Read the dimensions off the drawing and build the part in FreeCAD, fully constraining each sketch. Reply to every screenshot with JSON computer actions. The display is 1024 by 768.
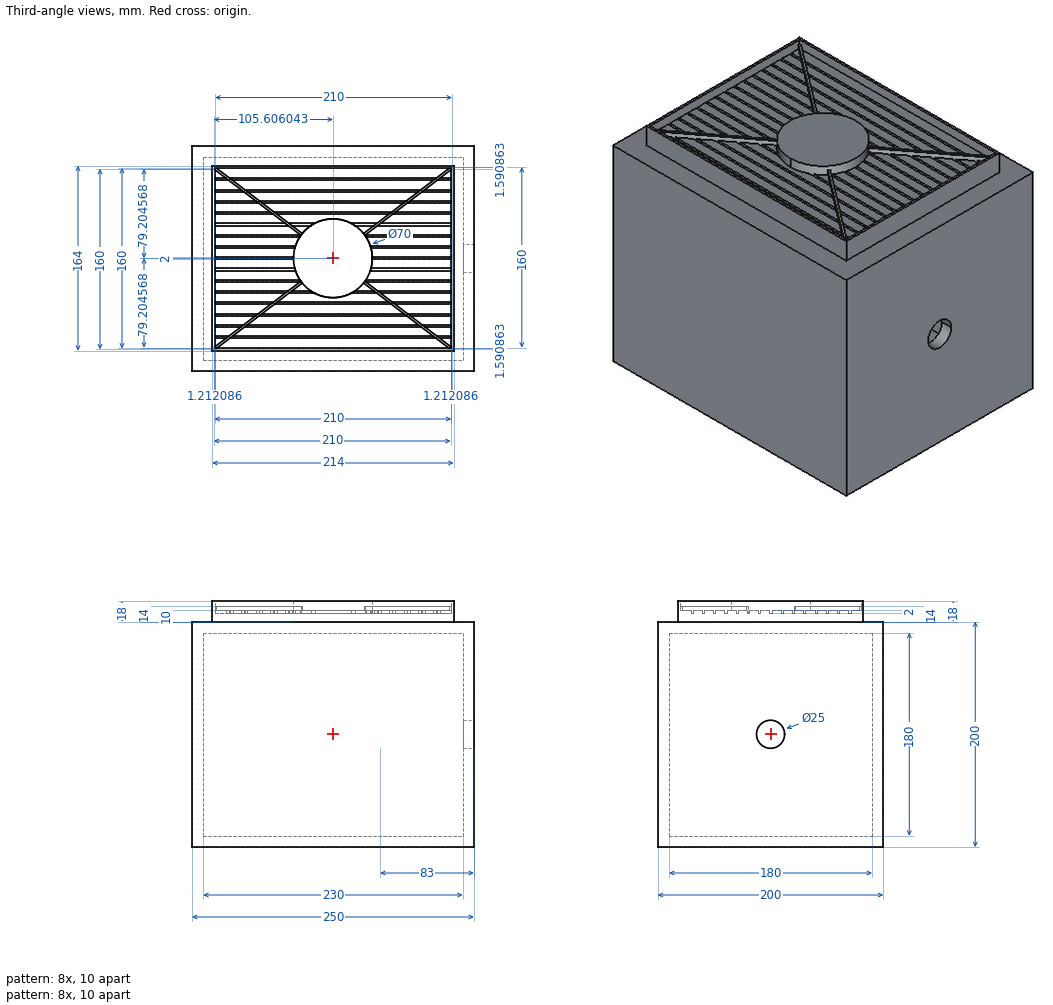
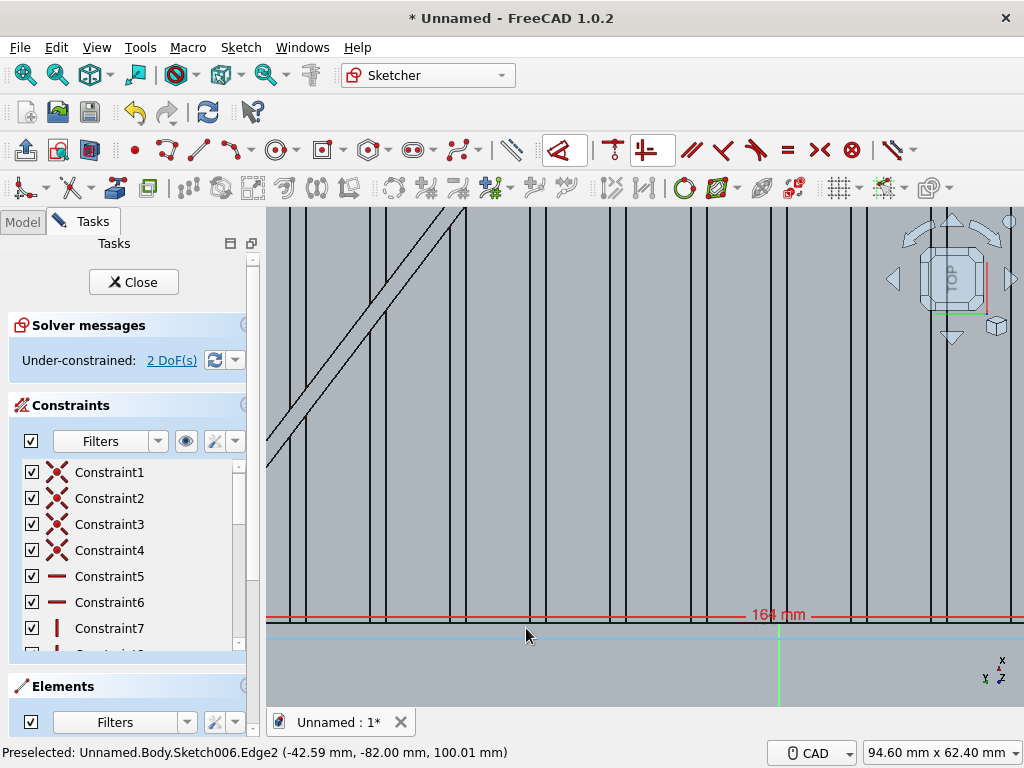
{"action": "left_click", "coordinate": [522, 622]}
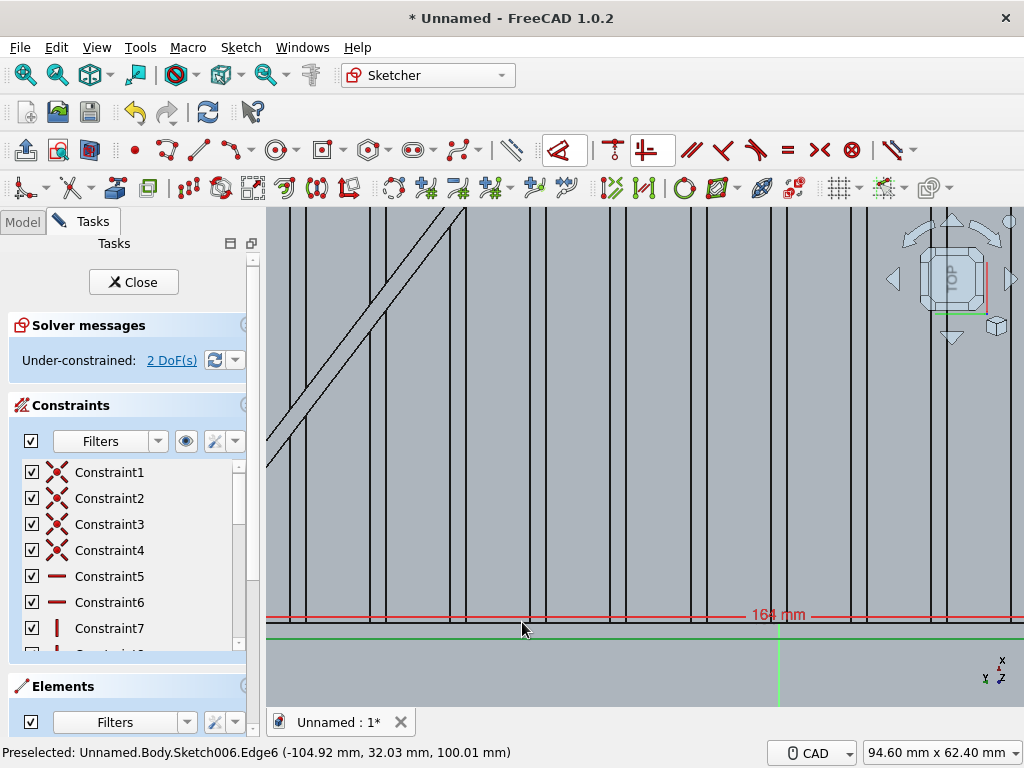
{"action": "left_click", "coordinate": [582, 150]}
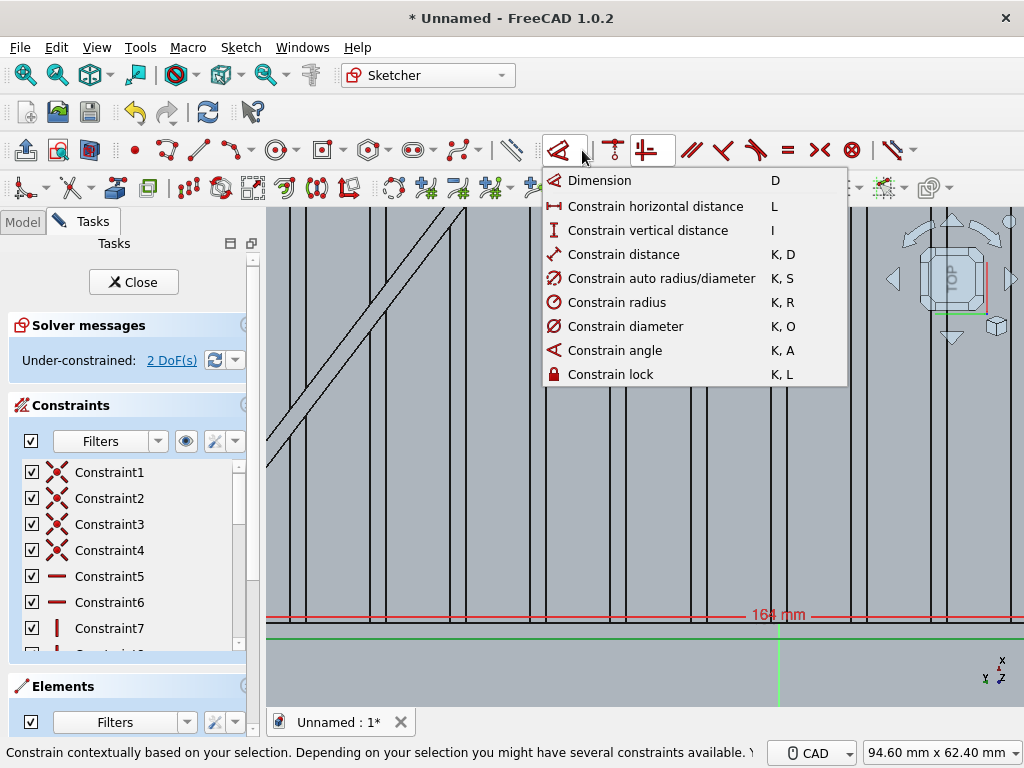
{"action": "left_click", "coordinate": [695, 206]}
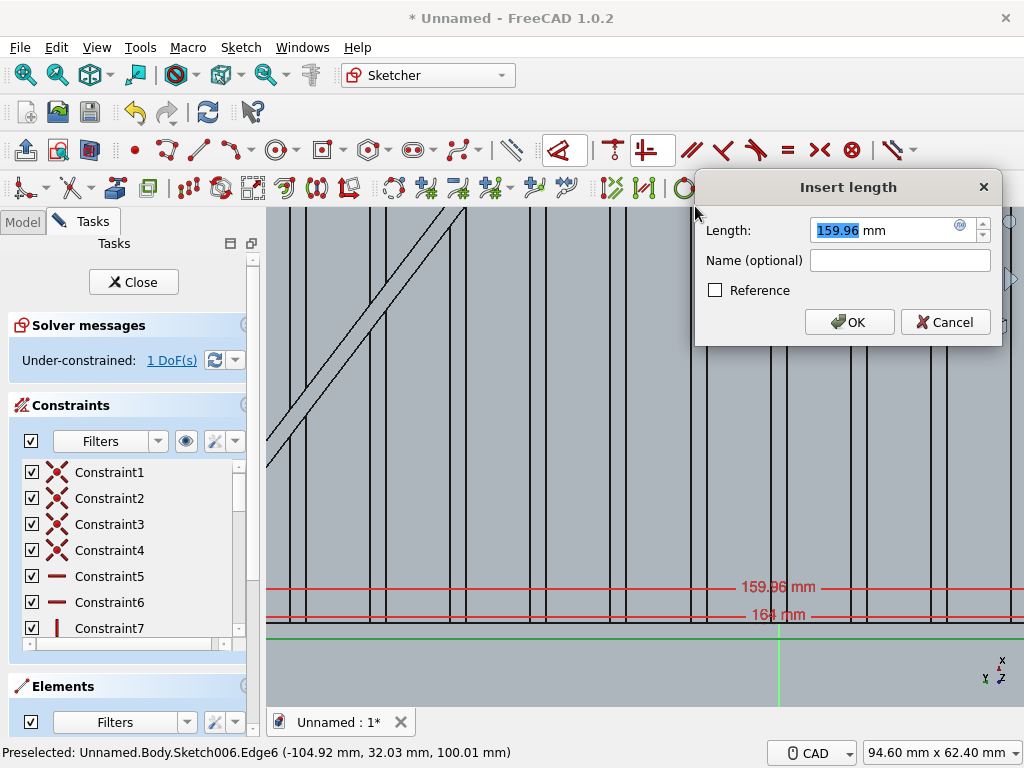
{"action": "type", "text": "160"}
{"action": "key", "text": "Return"}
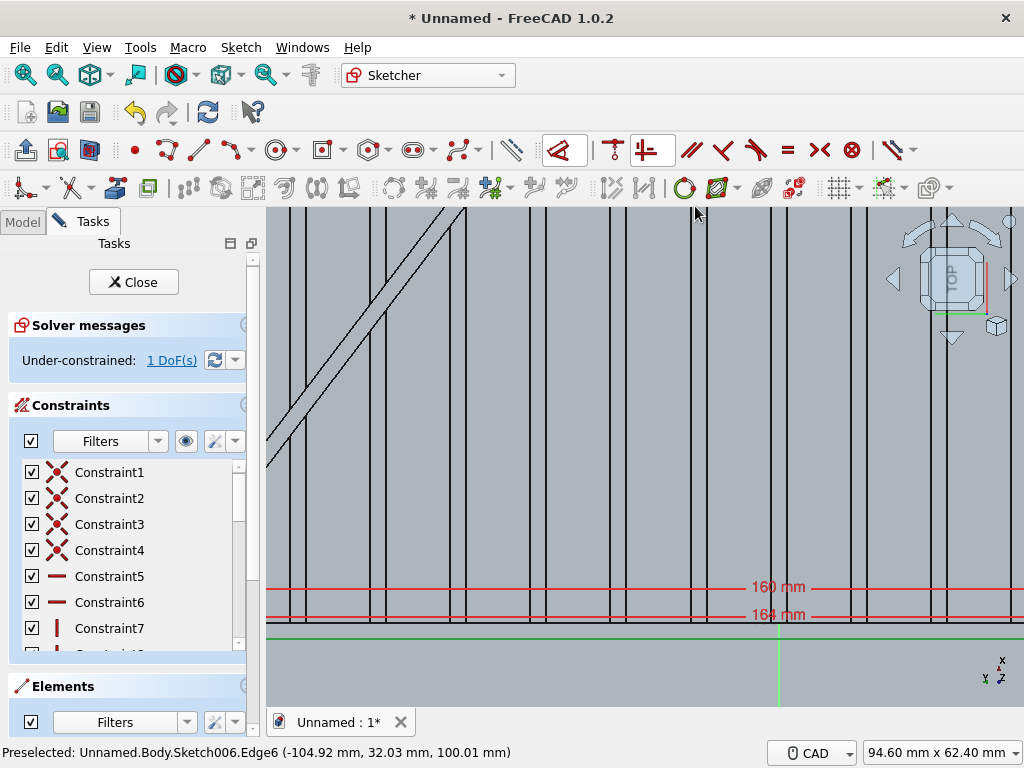
{"action": "scroll", "coordinate": [525, 628], "scroll_direction": "down", "scroll_amount": 8}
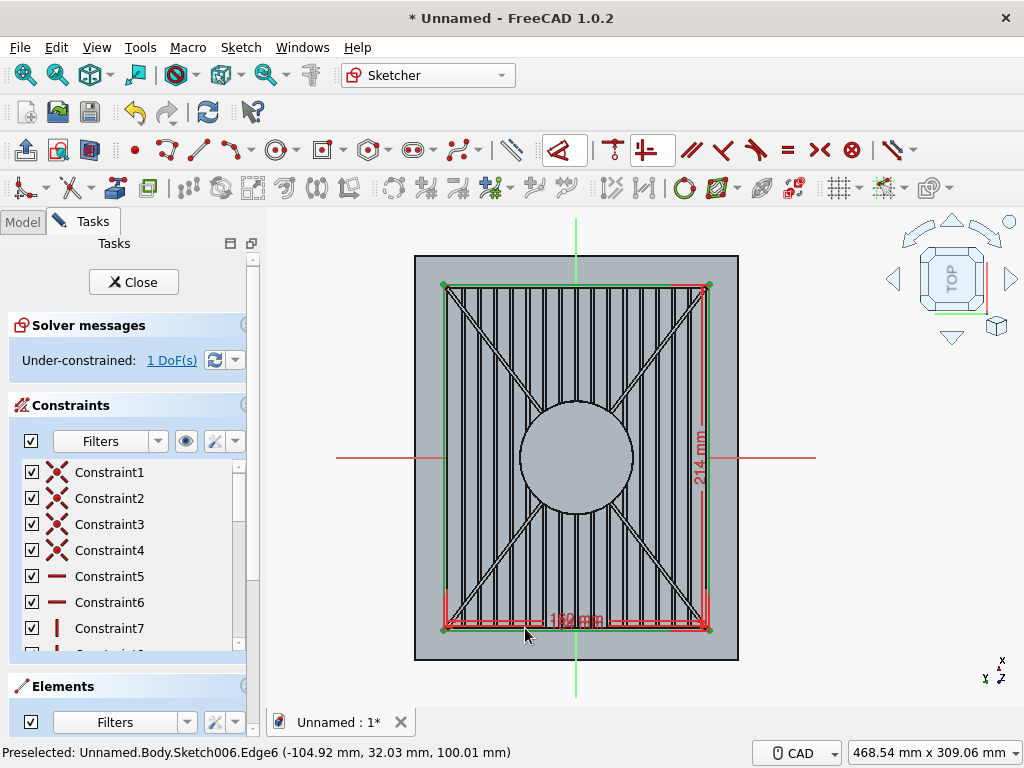
{"action": "scroll", "coordinate": [706, 526], "scroll_direction": "up", "scroll_amount": 8}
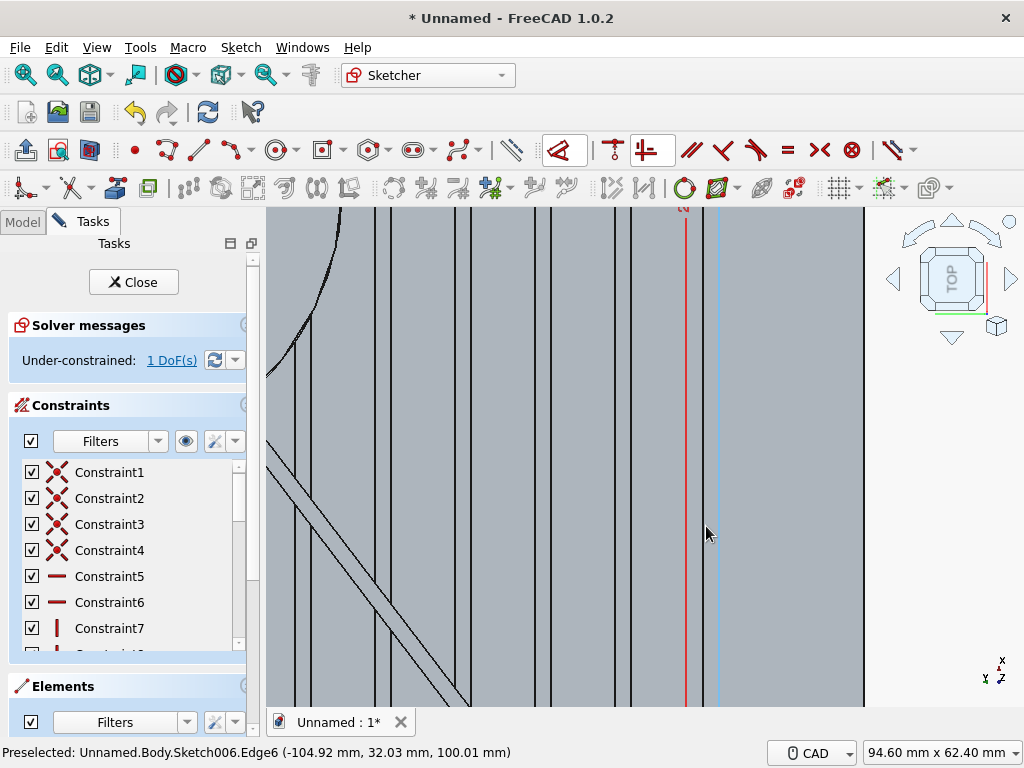
{"action": "left_click", "coordinate": [703, 522]}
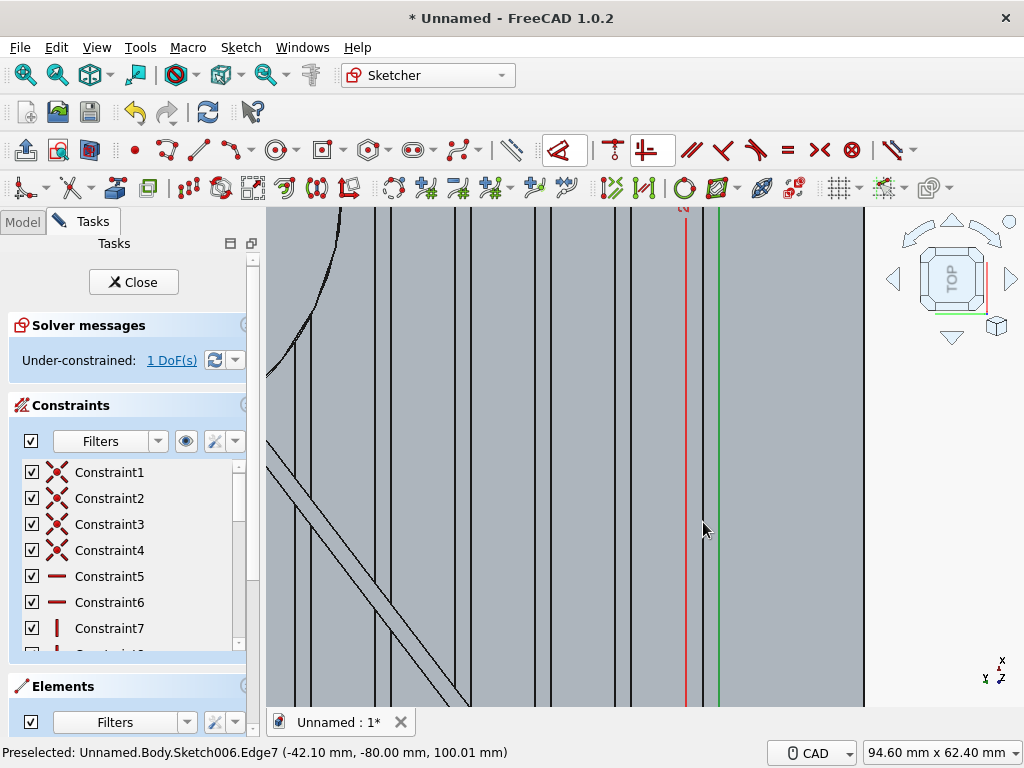
{"action": "key", "text": "i"}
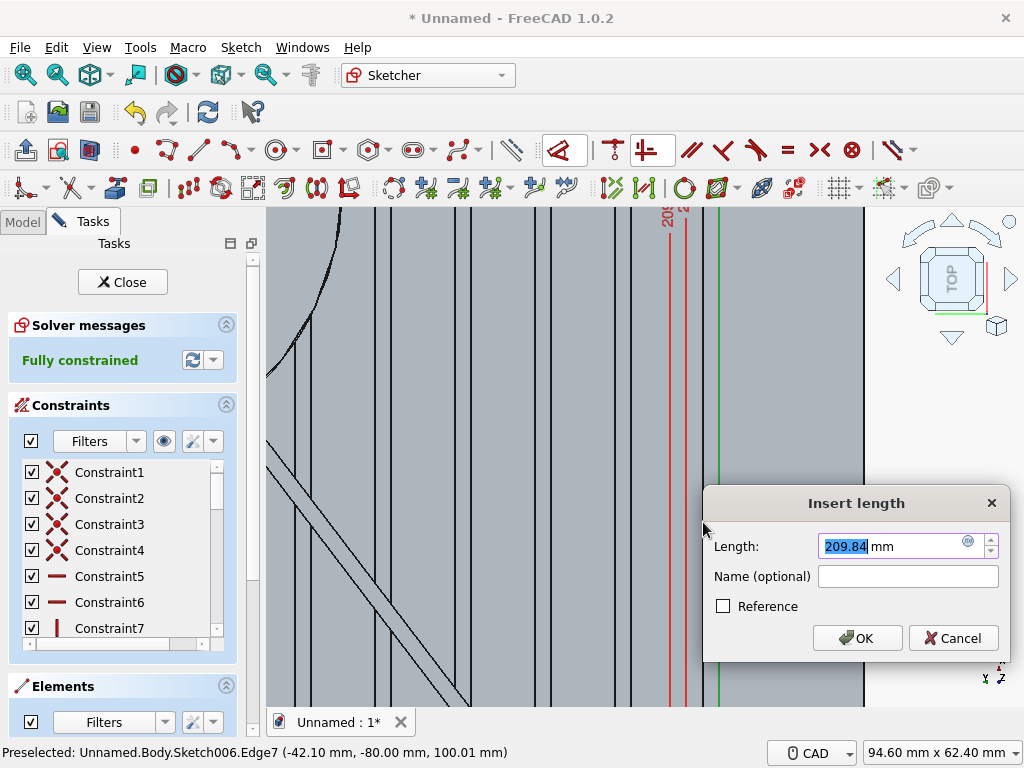
{"action": "type", "text": "210"}
{"action": "key", "text": "Return"}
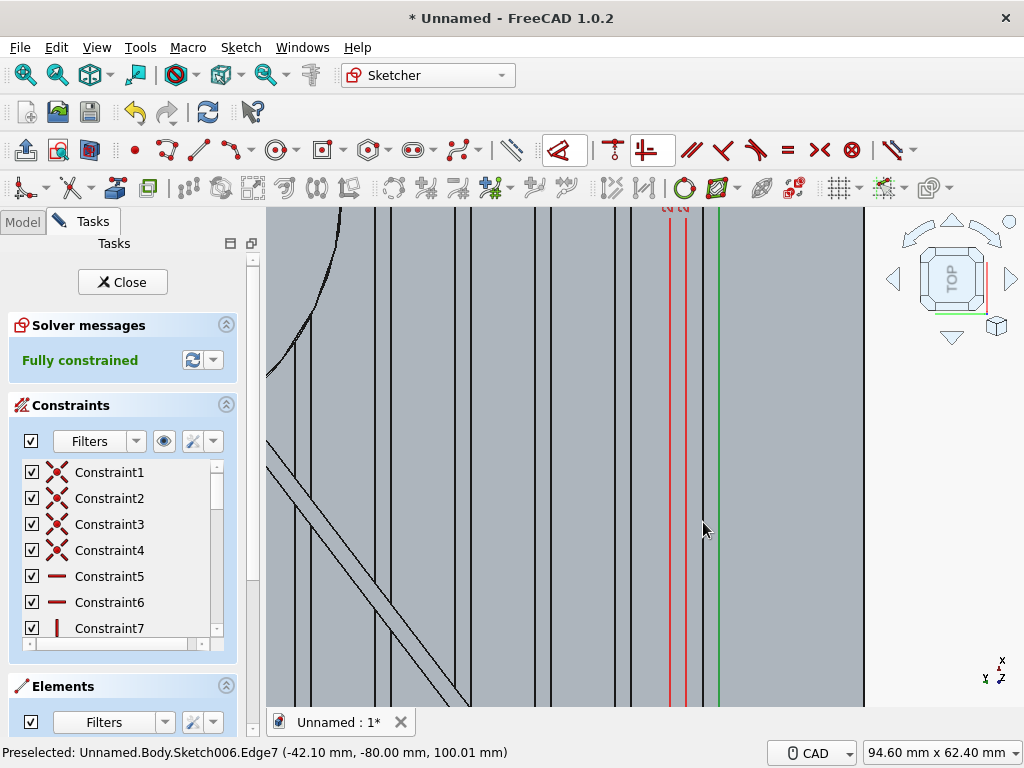
{"action": "left_click", "coordinate": [123, 282]}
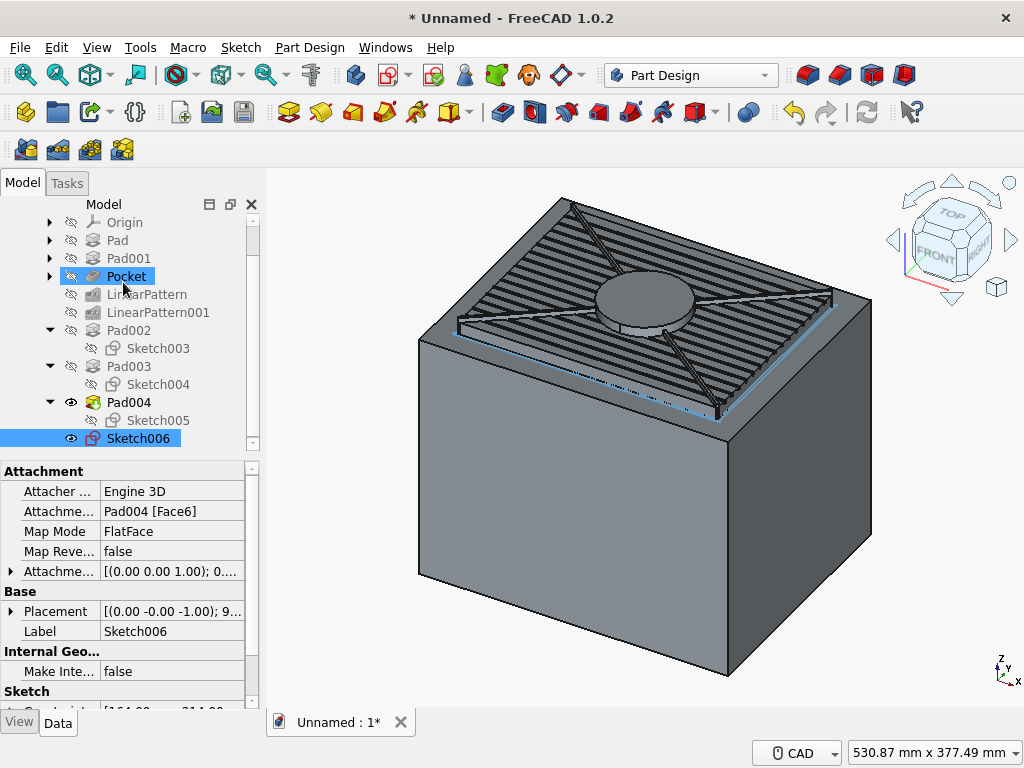
{"action": "left_click", "coordinate": [290, 112]}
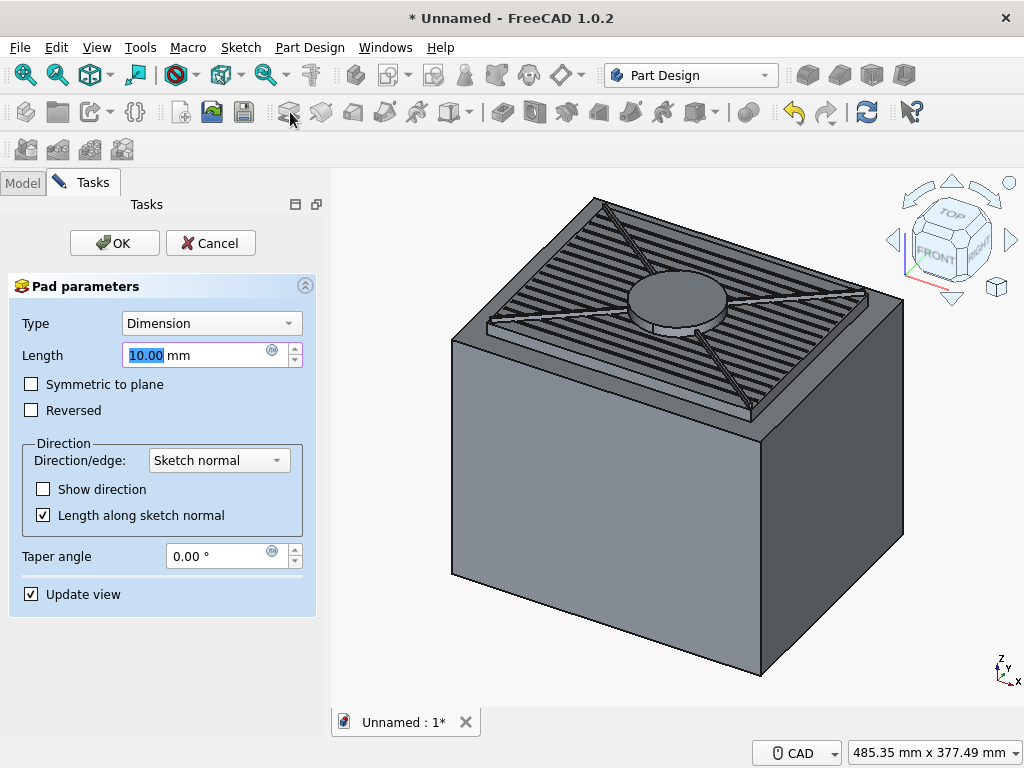
{"action": "type", "text": "18"}
{"action": "key", "text": "Tab"}